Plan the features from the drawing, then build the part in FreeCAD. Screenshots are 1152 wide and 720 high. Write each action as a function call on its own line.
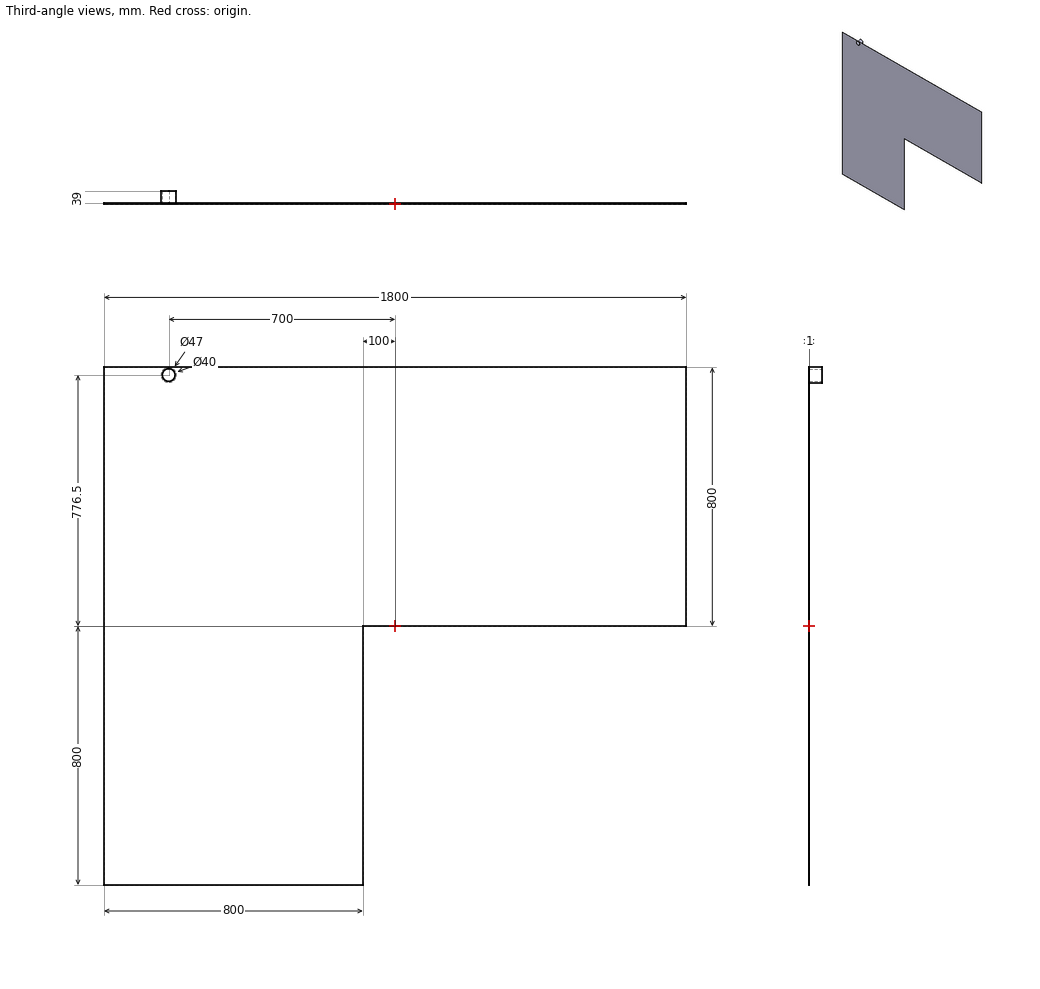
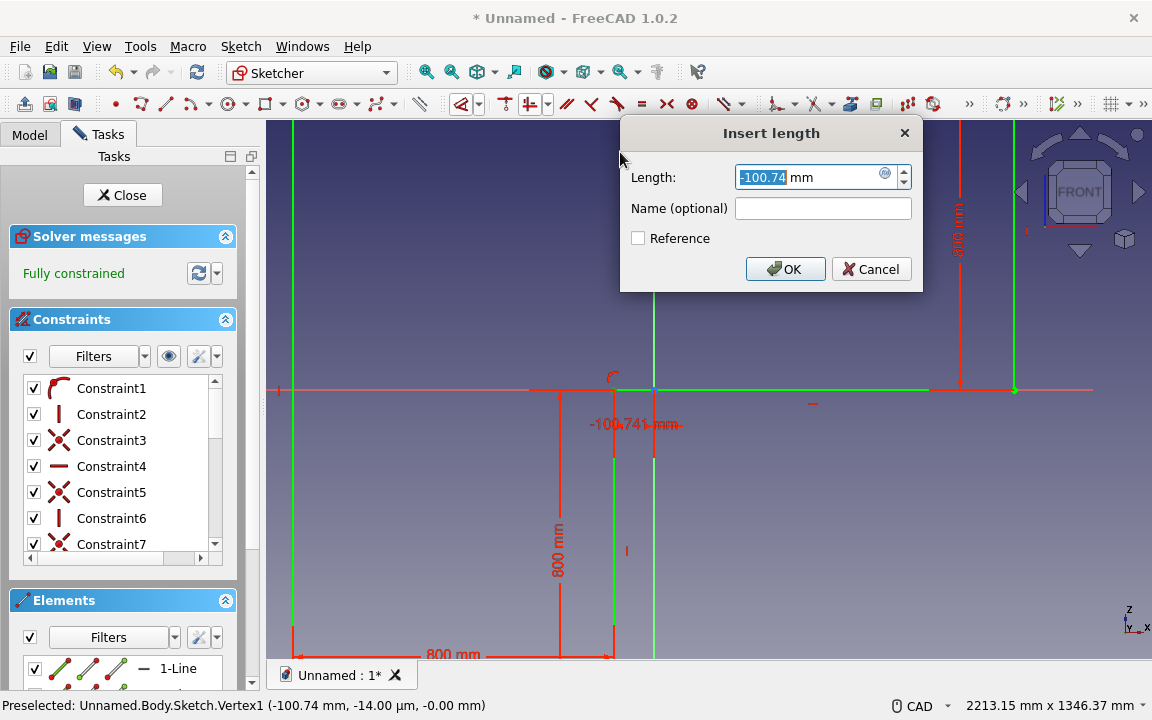
text(-100)
key(Return)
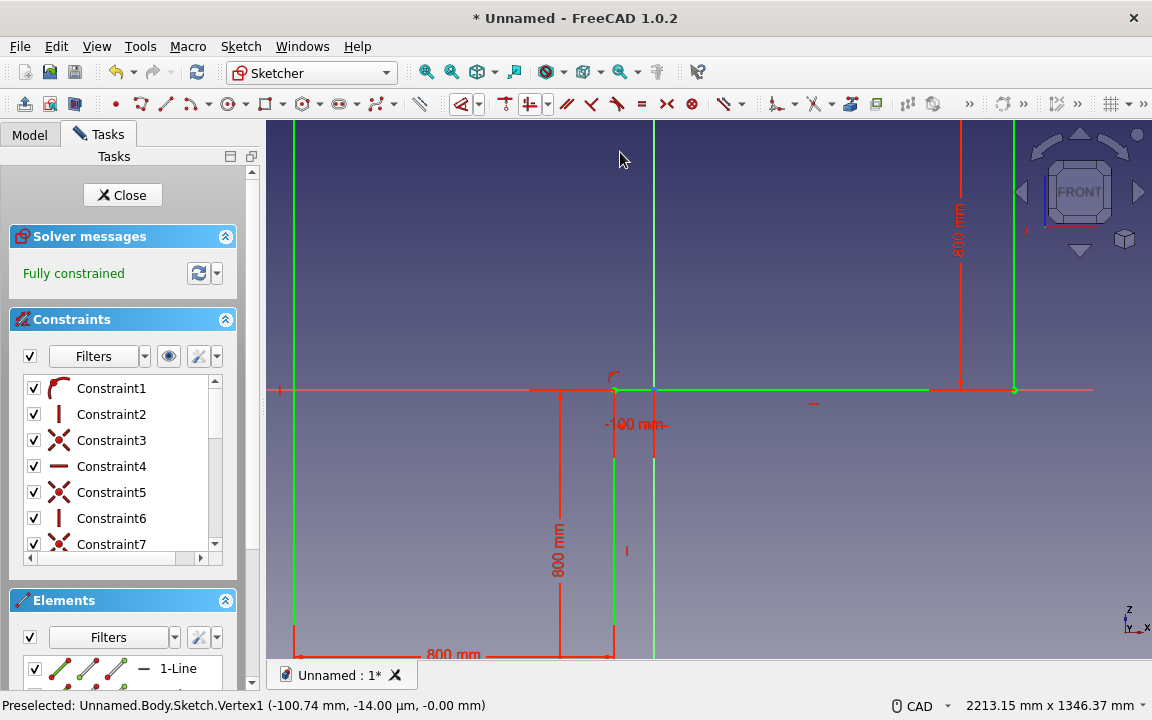
click(123, 195)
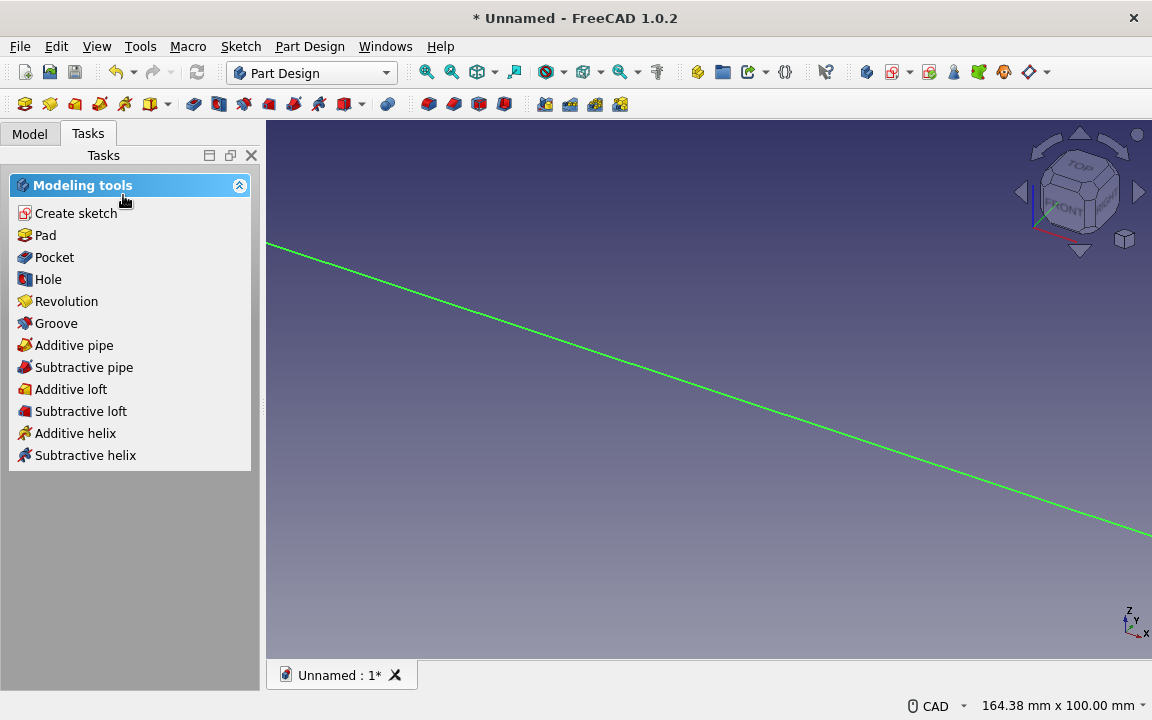
click(25, 104)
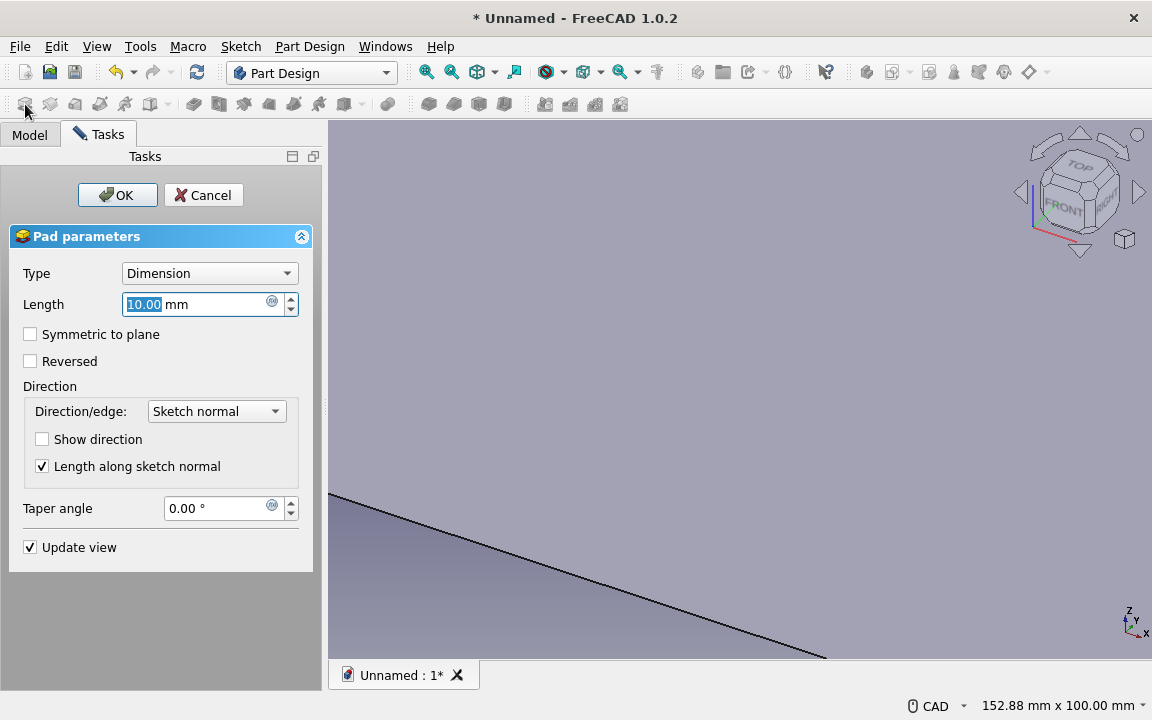
text(1)
key(Tab)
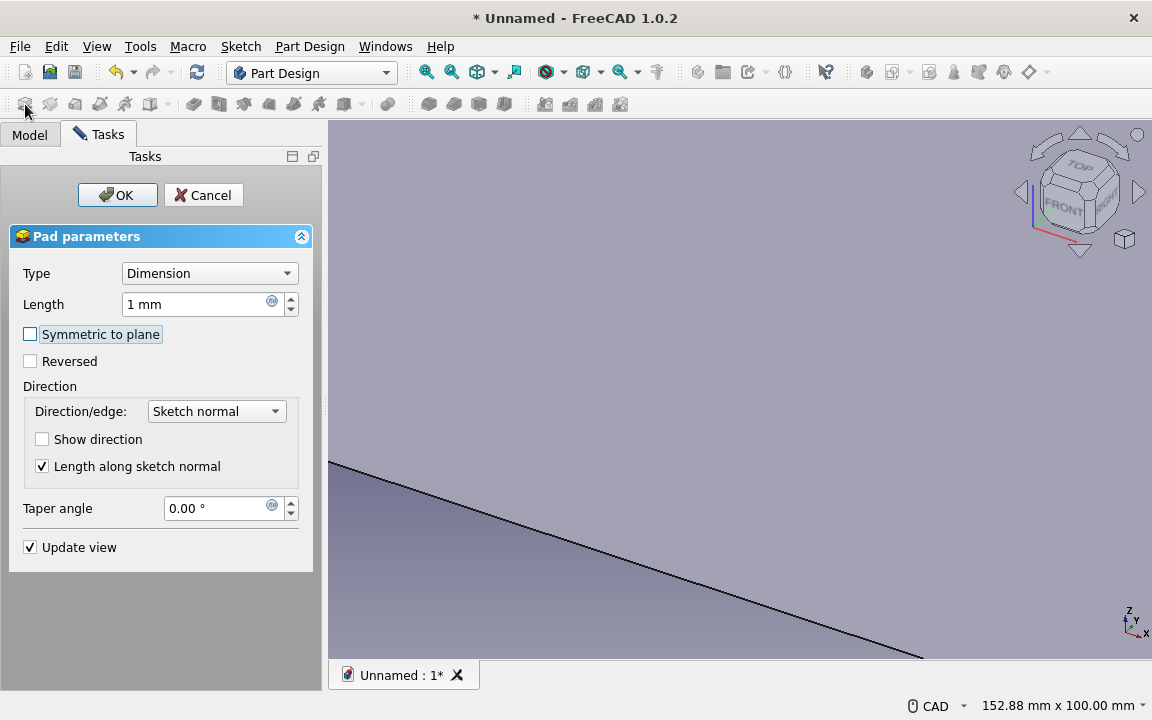
click(31, 361)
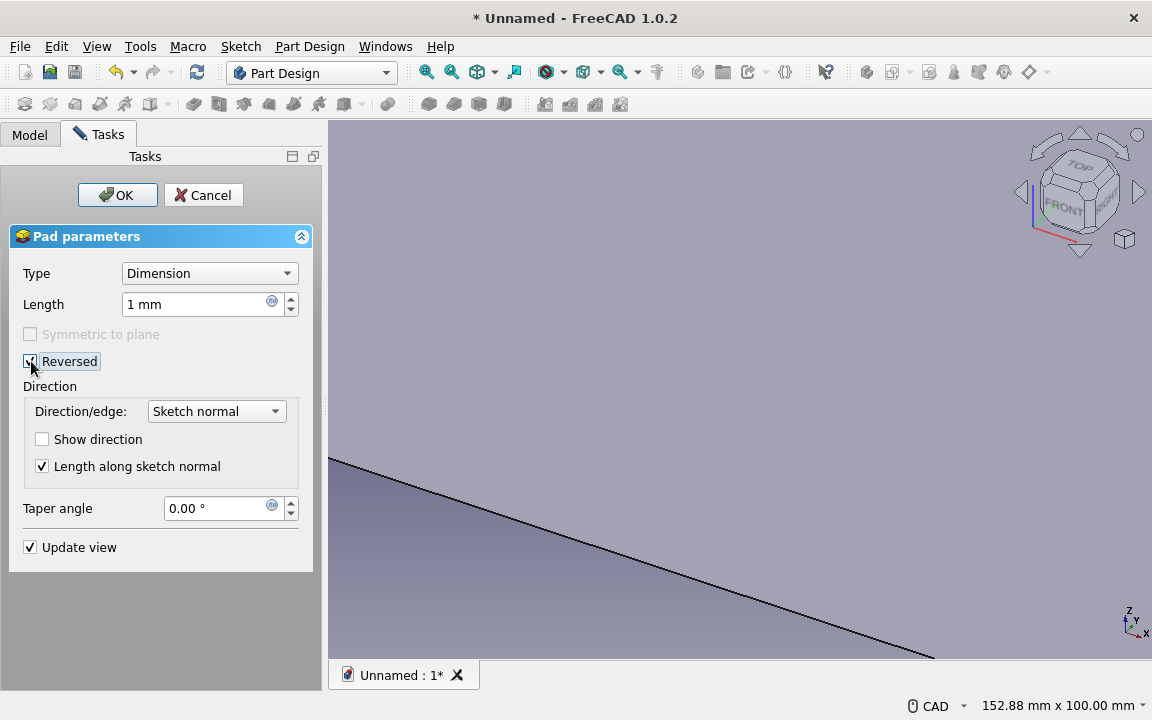
click(118, 195)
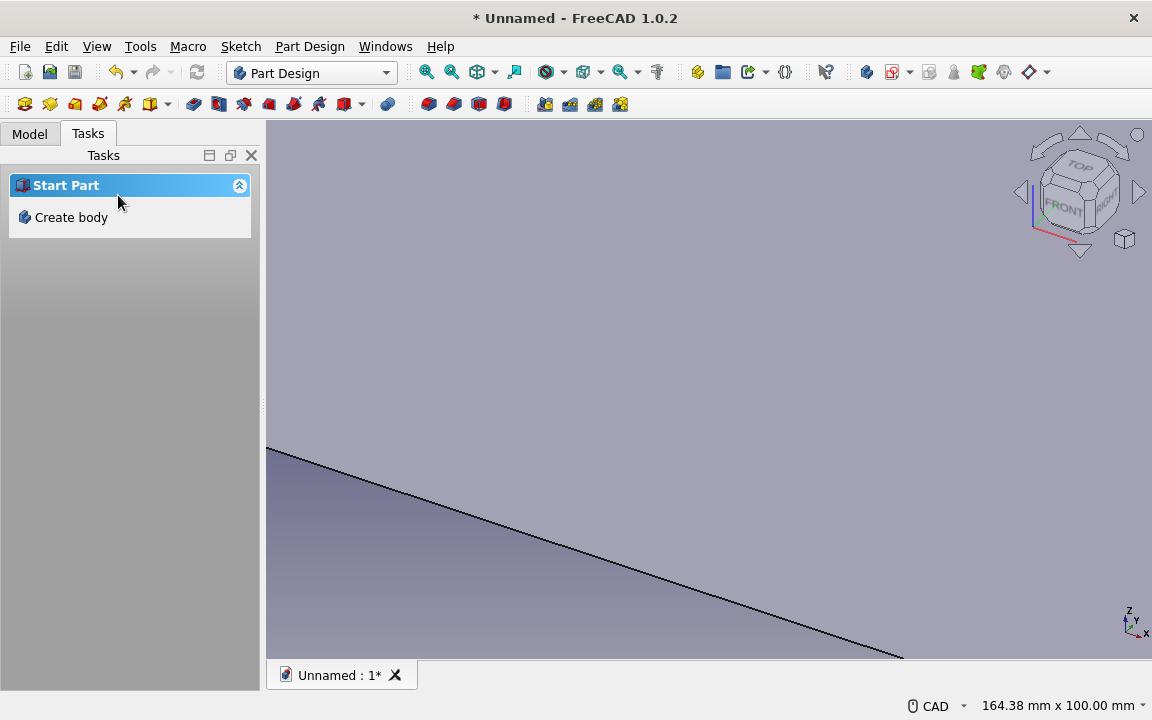
click(427, 72)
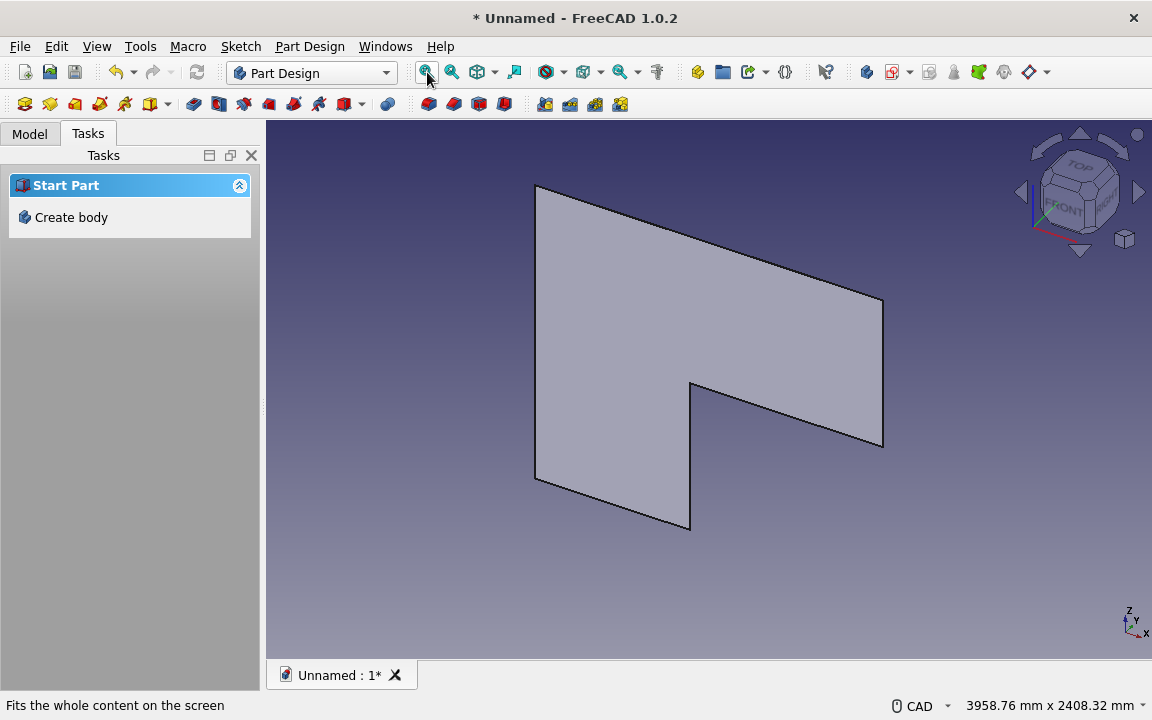
key(4)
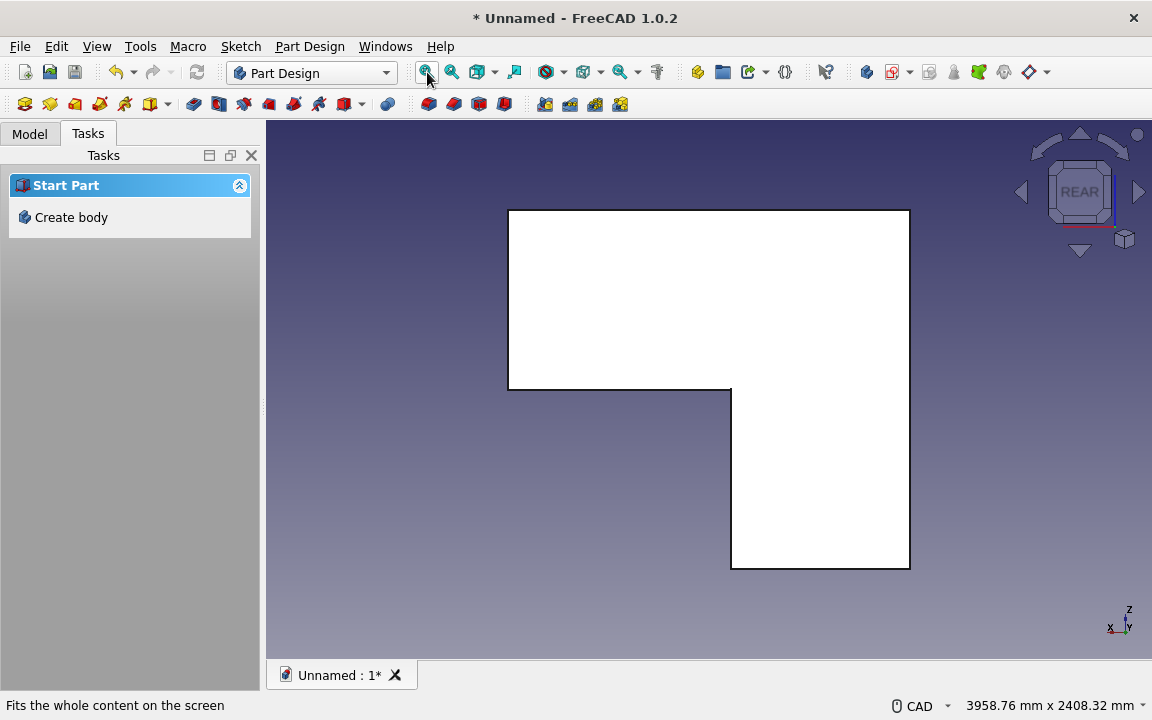
click(824, 337)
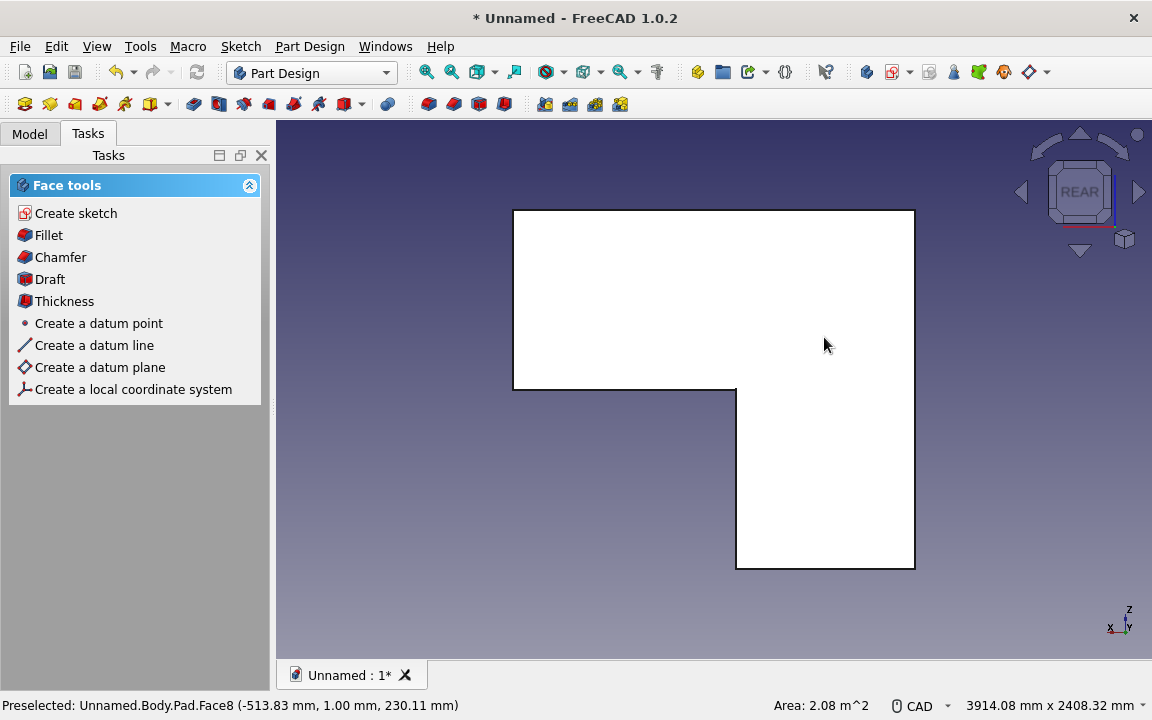
click(892, 72)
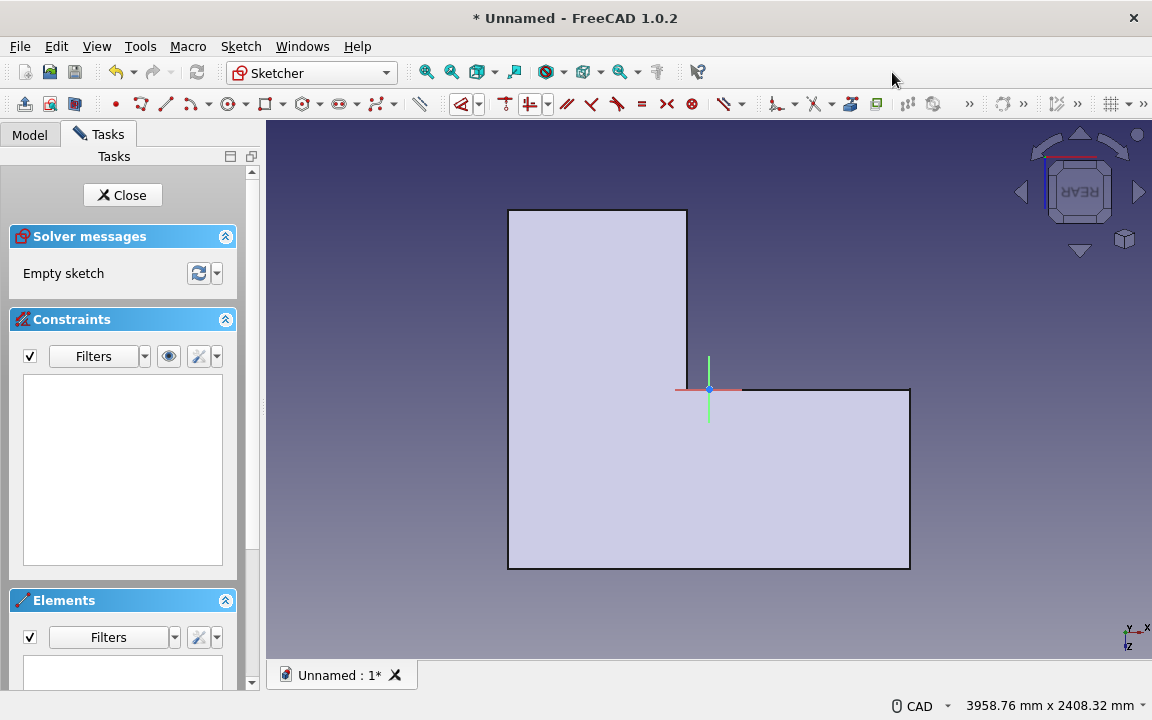
scroll(548, 572, up, 15)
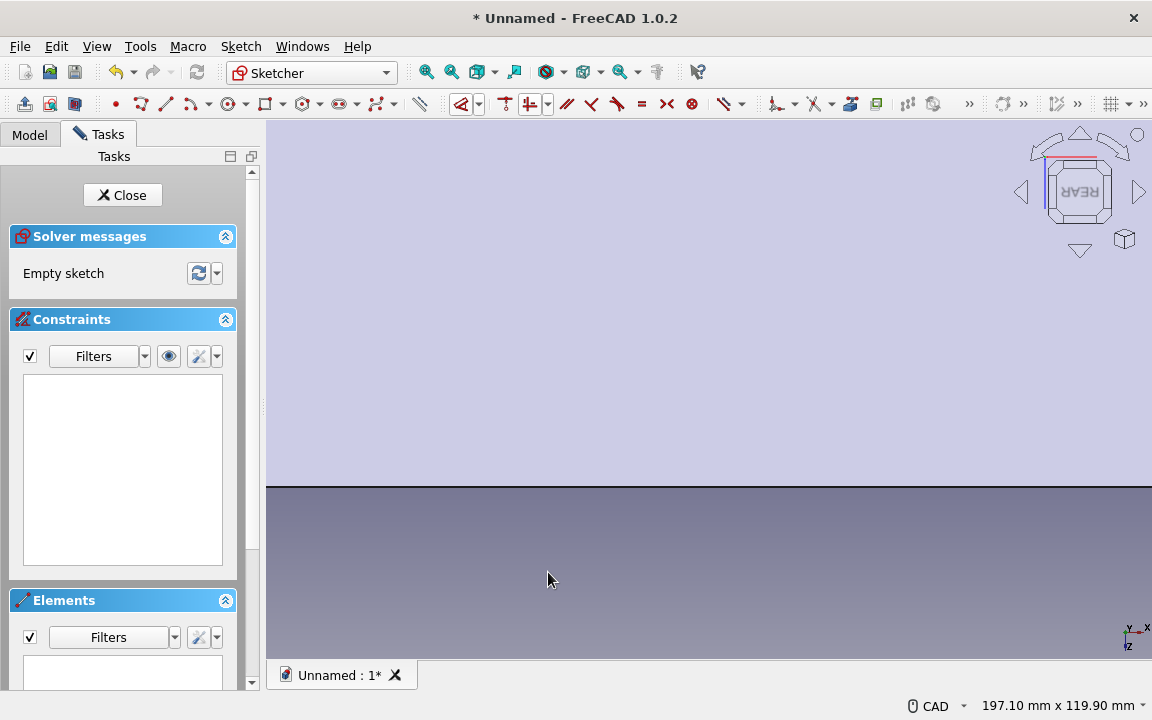
scroll(615, 371, up, 3)